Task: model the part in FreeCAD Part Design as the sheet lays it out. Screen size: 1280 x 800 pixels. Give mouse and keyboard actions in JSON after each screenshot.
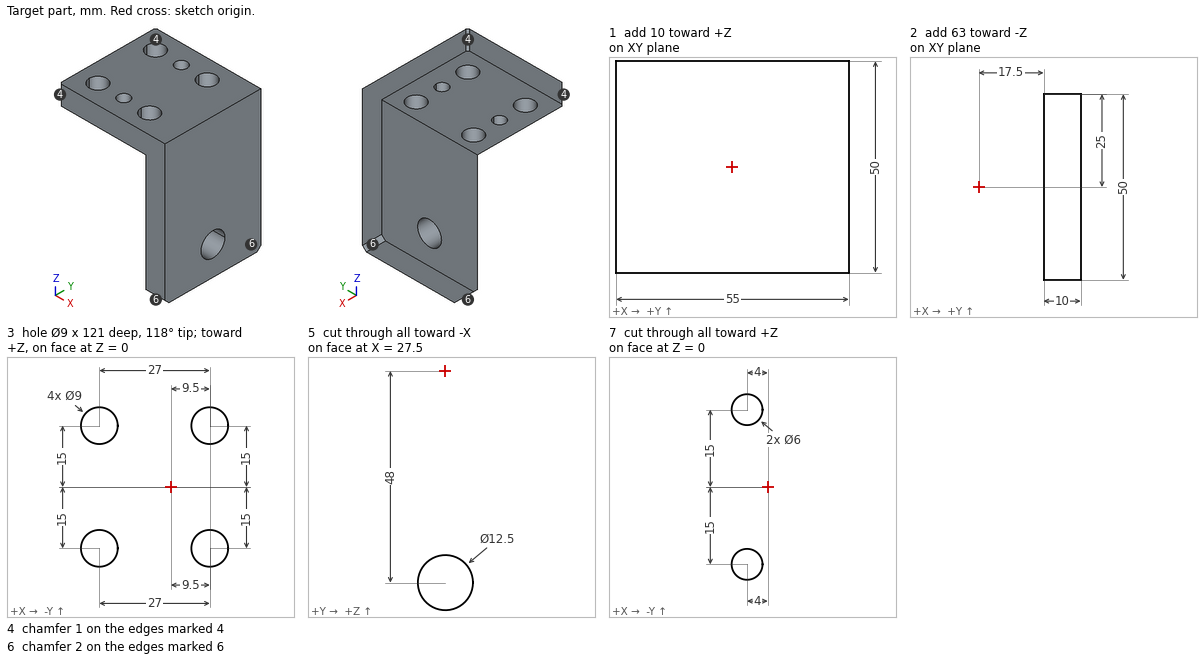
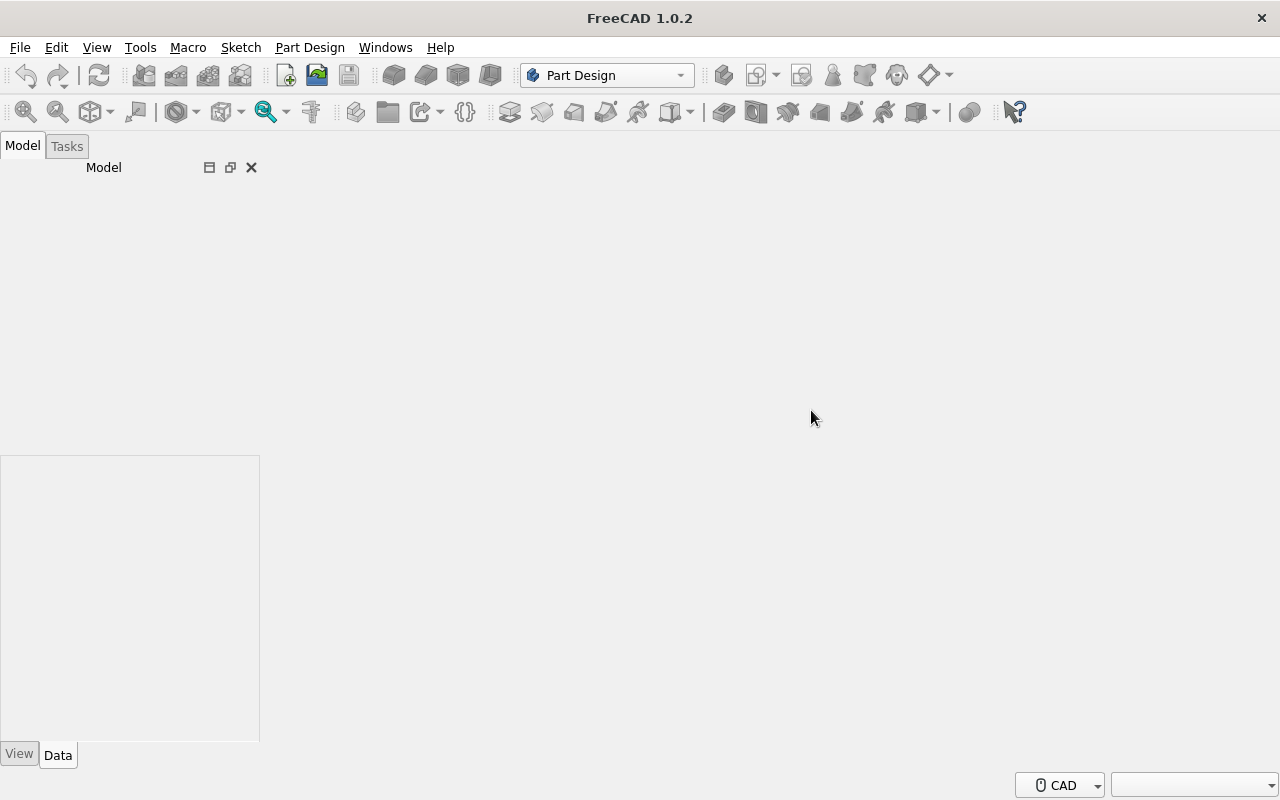
{"action": "left_click", "coordinate": [286, 76]}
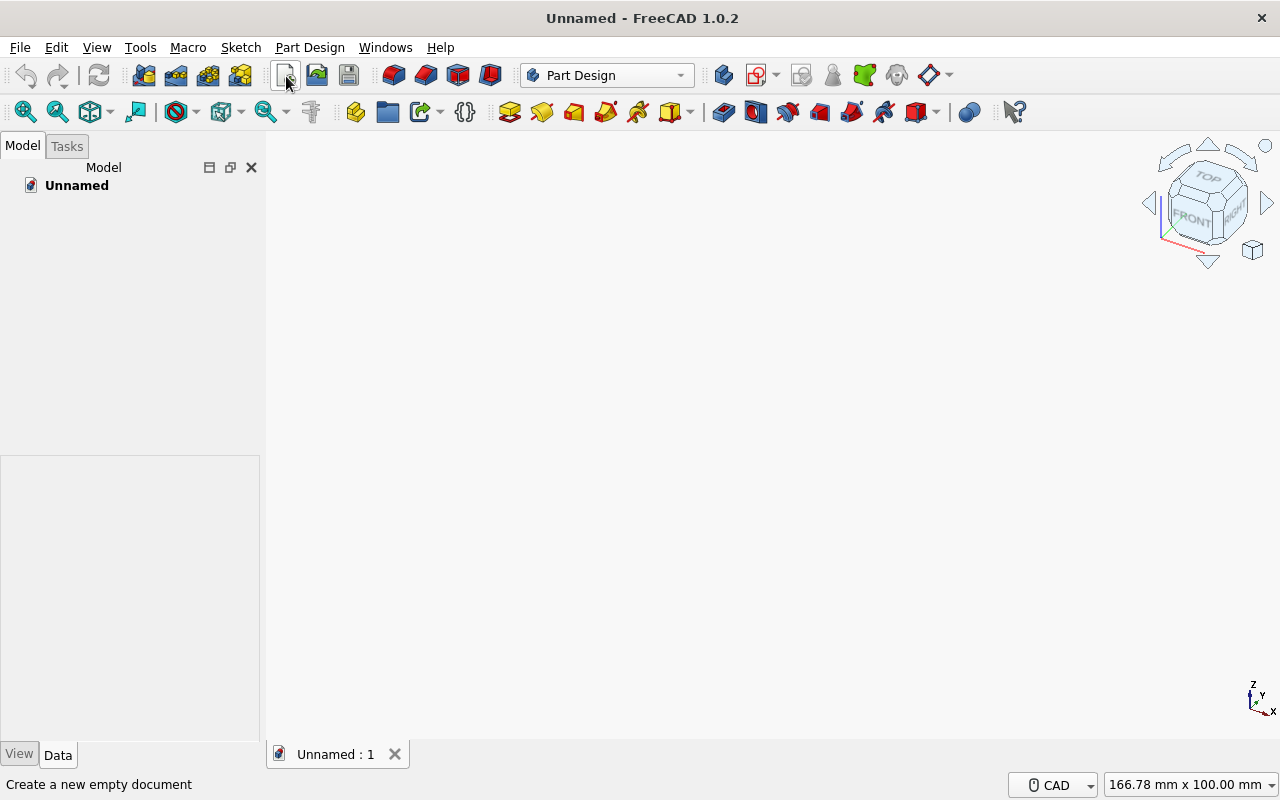
{"action": "left_click", "coordinate": [756, 76]}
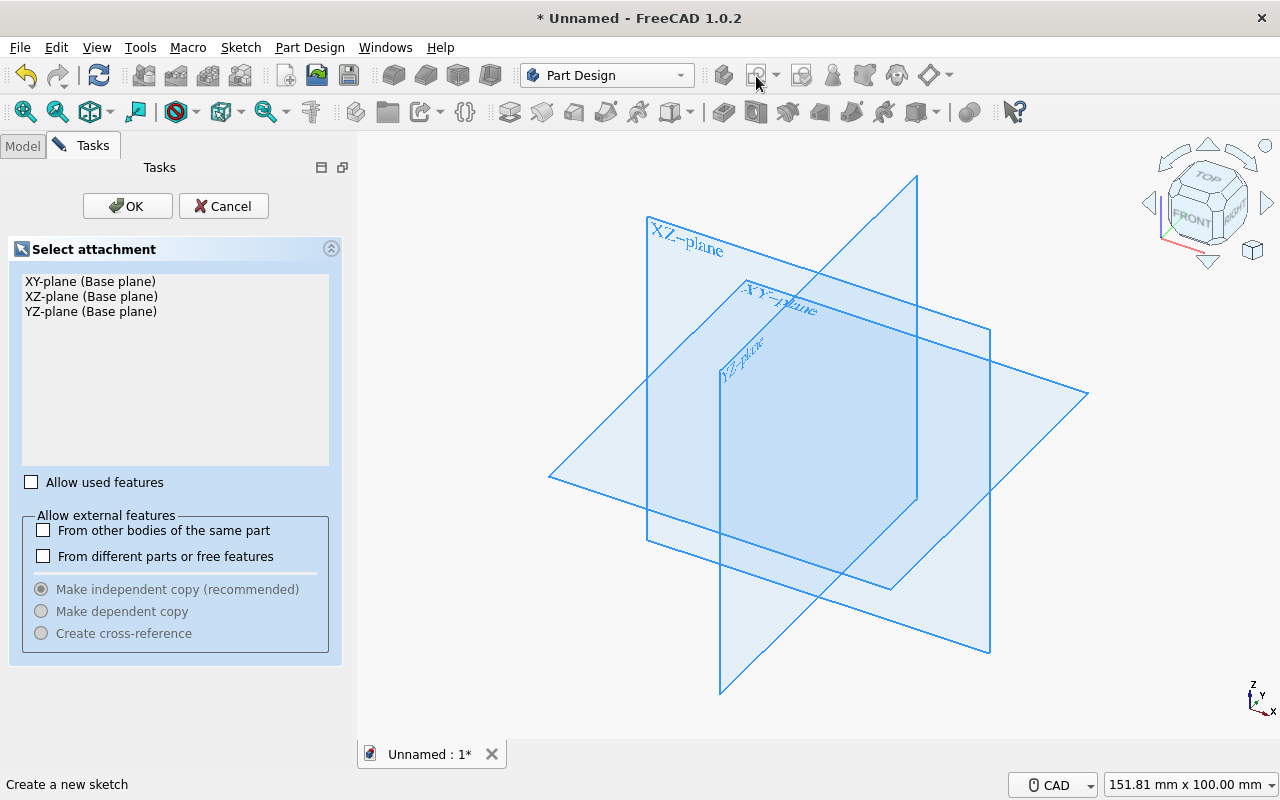
{"action": "left_click", "coordinate": [82, 282]}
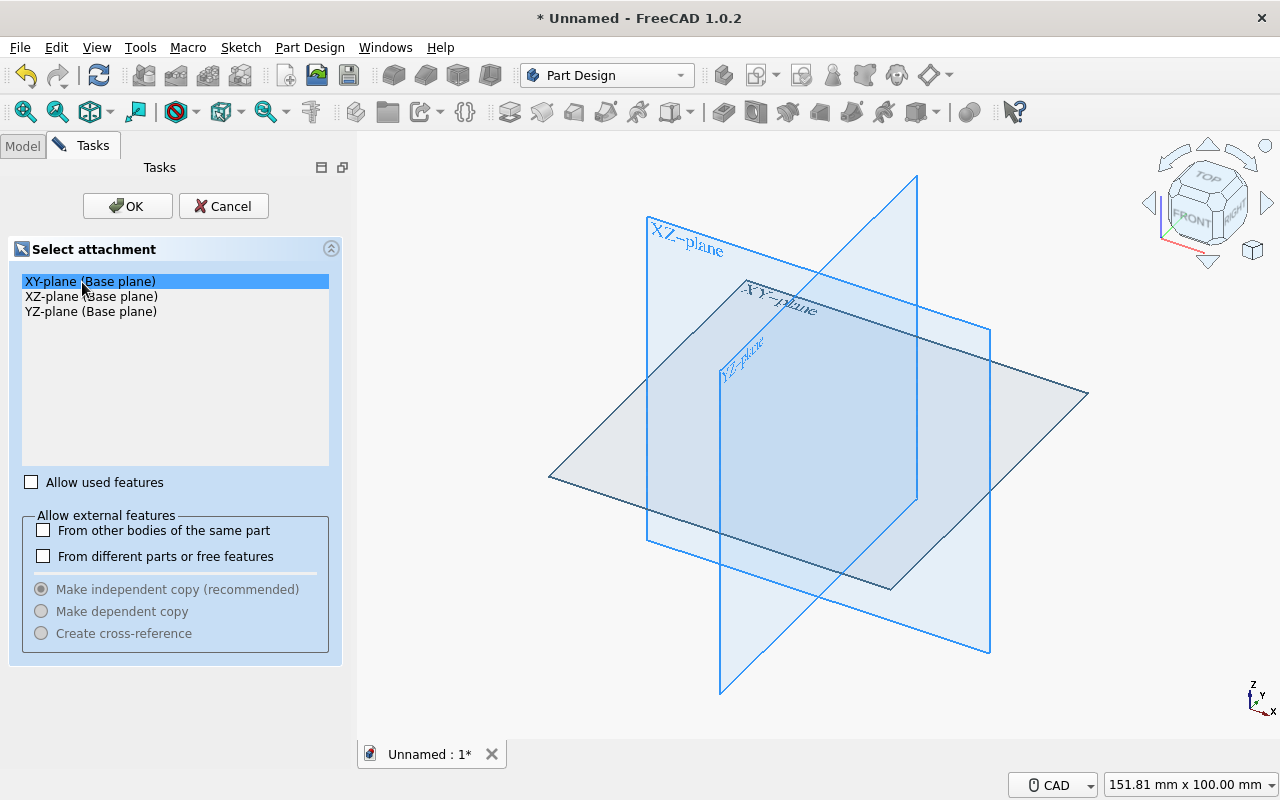
{"action": "left_click", "coordinate": [128, 206]}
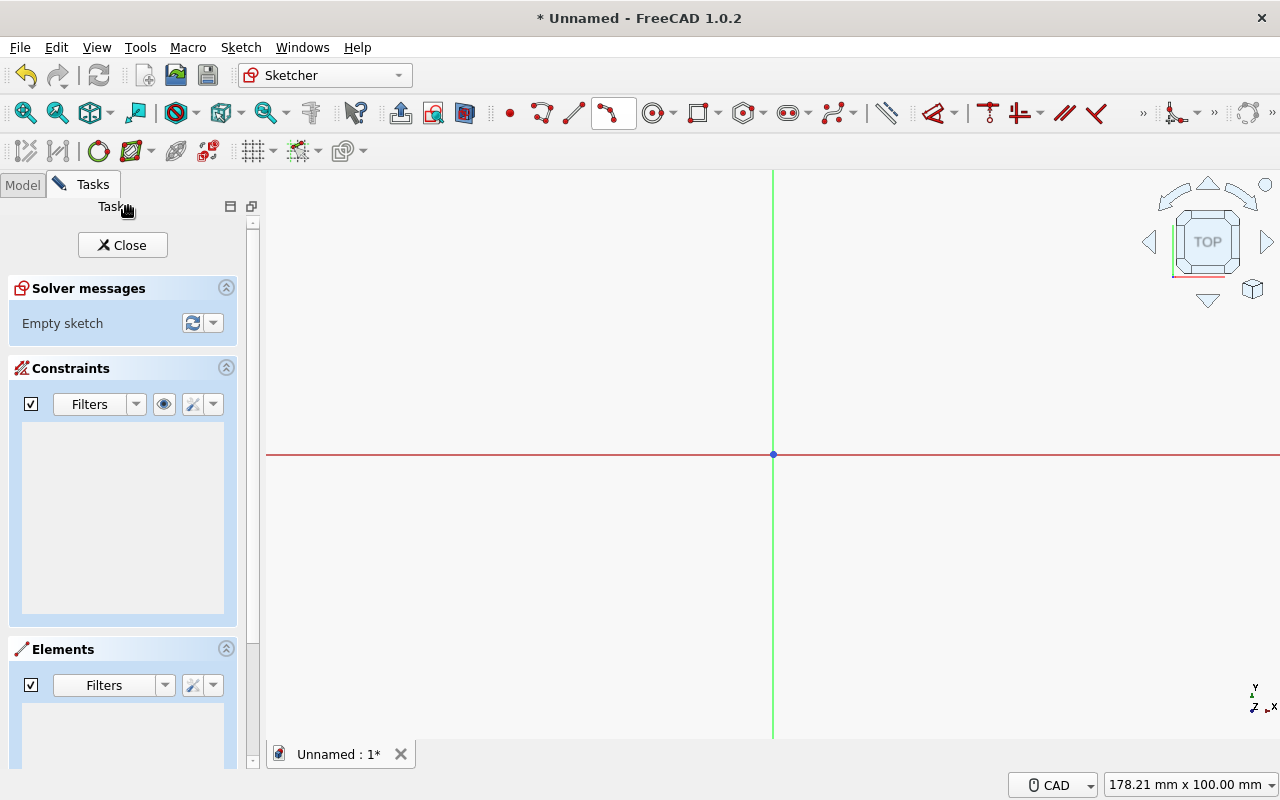
{"action": "left_click", "coordinate": [720, 114]}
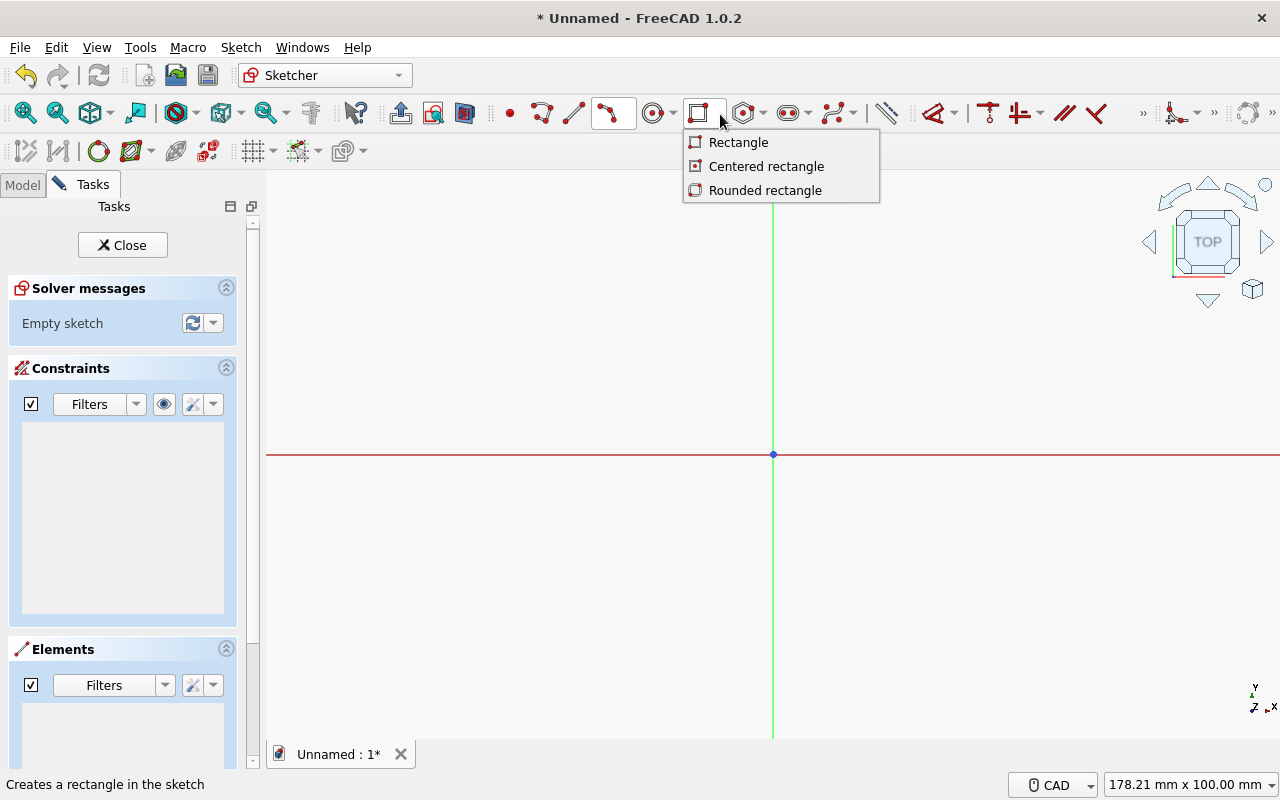
{"action": "left_click", "coordinate": [782, 166]}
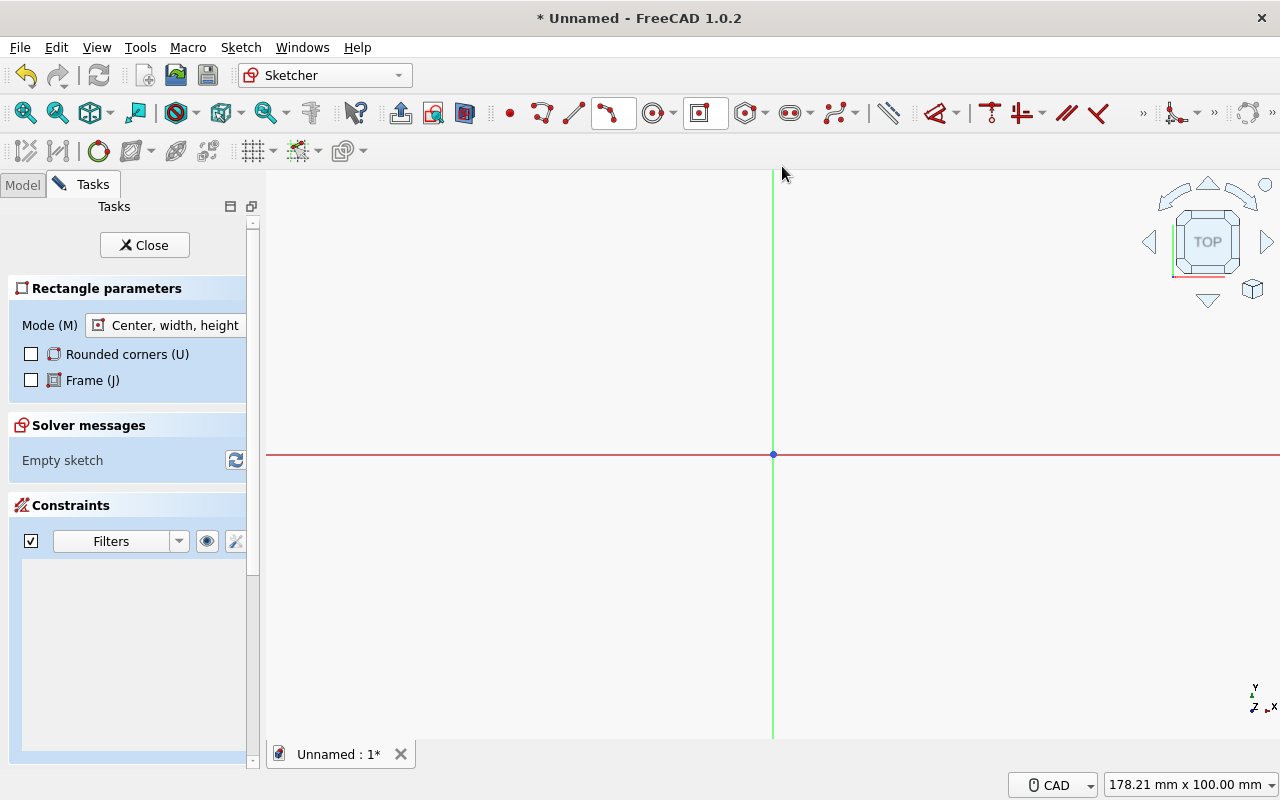
{"action": "left_click", "coordinate": [773, 454]}
{"action": "left_click", "coordinate": [929, 312]}
{"action": "key", "text": "Escape"}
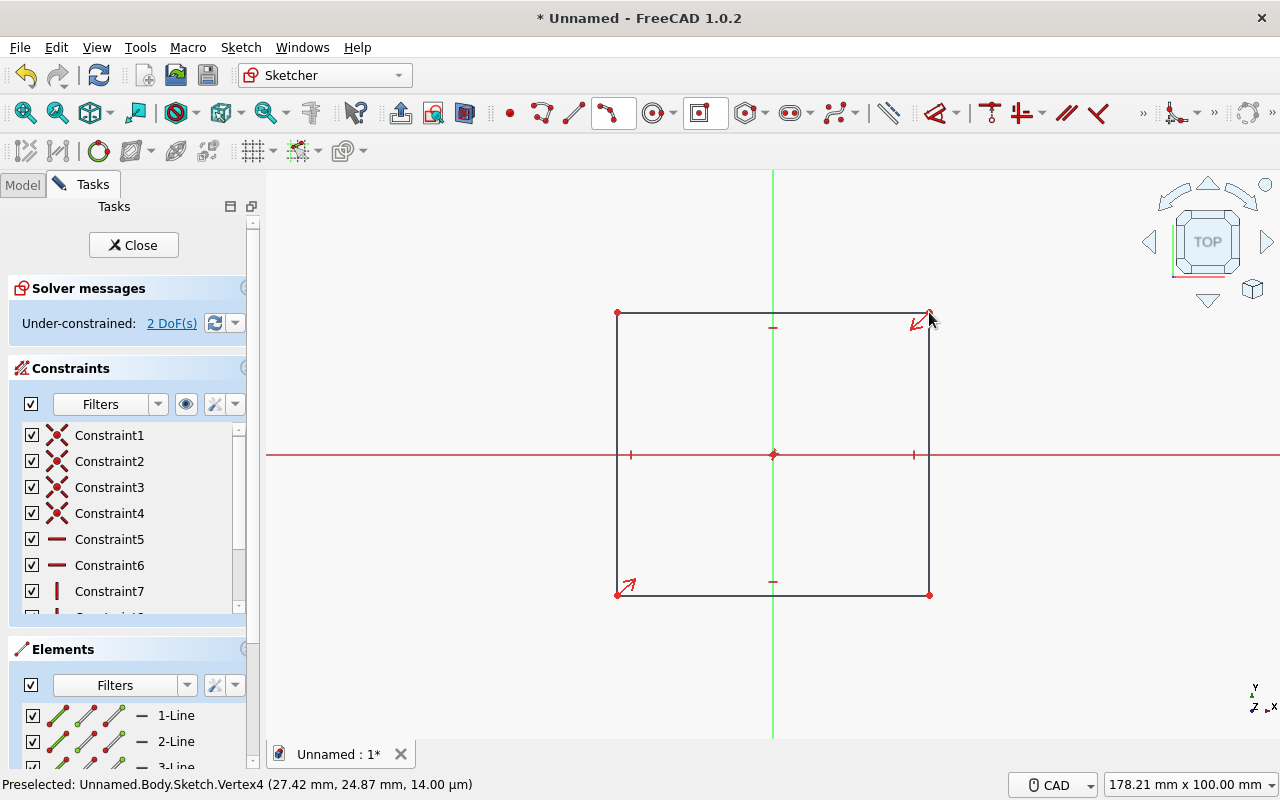
{"action": "key", "text": "d"}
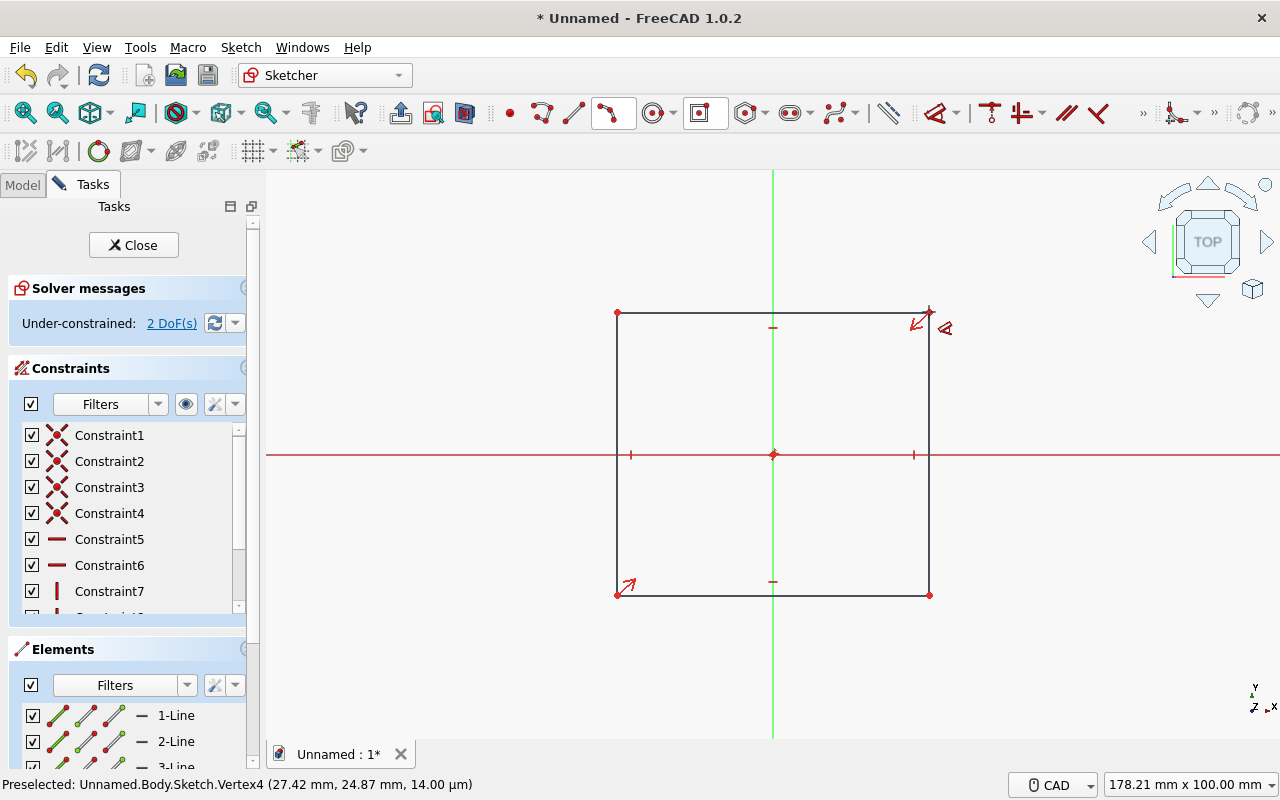
{"action": "left_click", "coordinate": [711, 596]}
{"action": "left_click", "coordinate": [701, 630]}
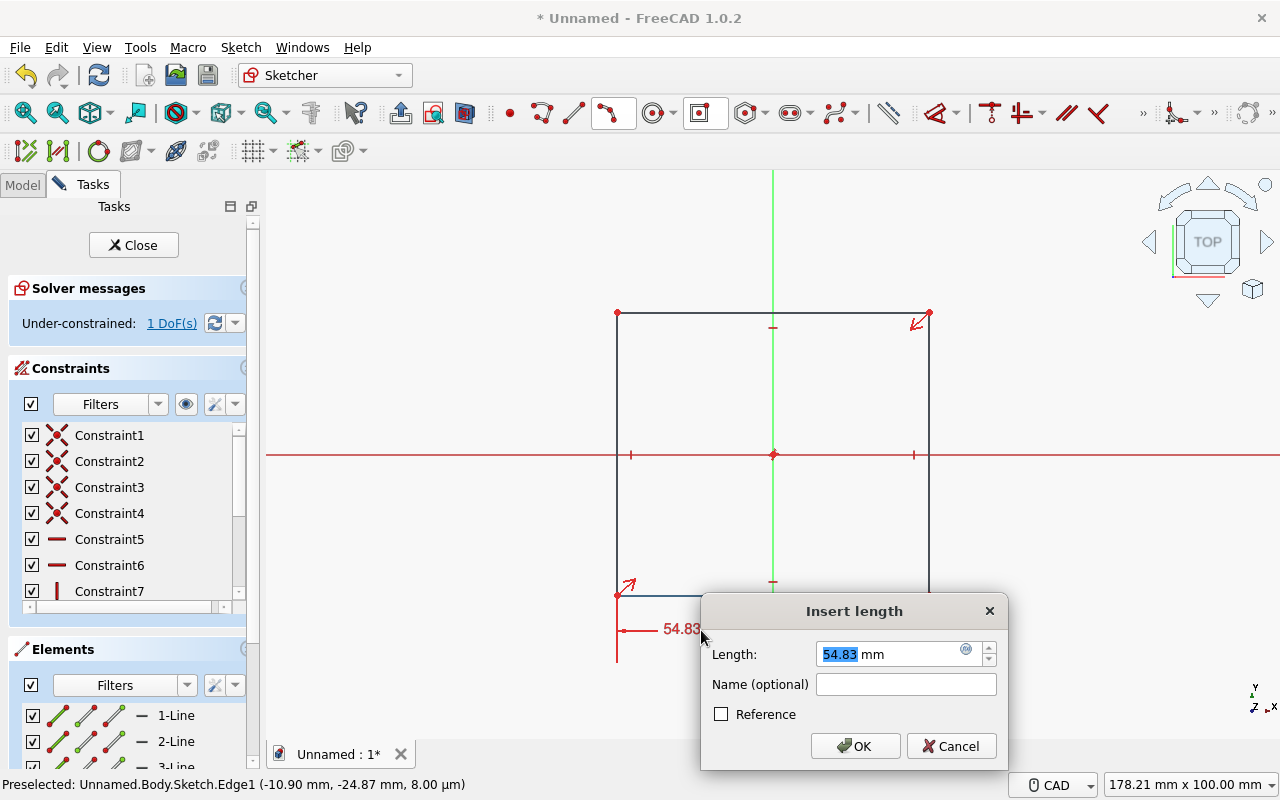
{"action": "type", "text": "55"}
{"action": "key", "text": "Return"}